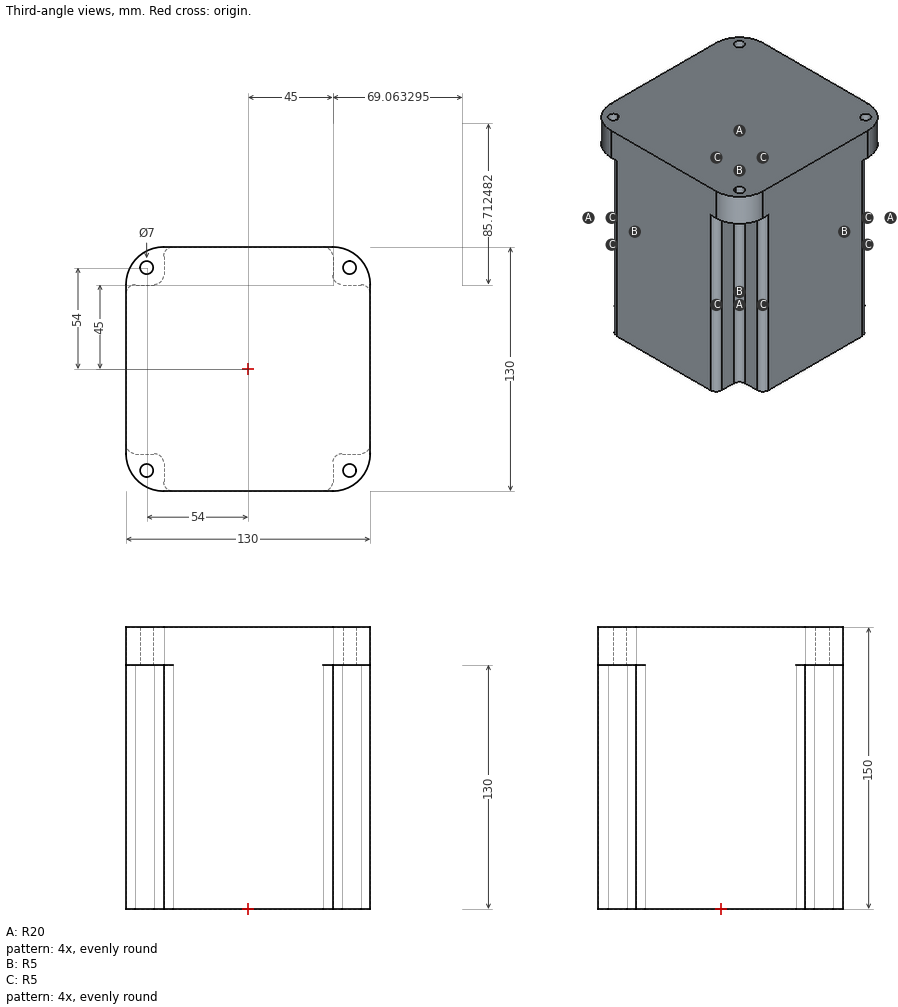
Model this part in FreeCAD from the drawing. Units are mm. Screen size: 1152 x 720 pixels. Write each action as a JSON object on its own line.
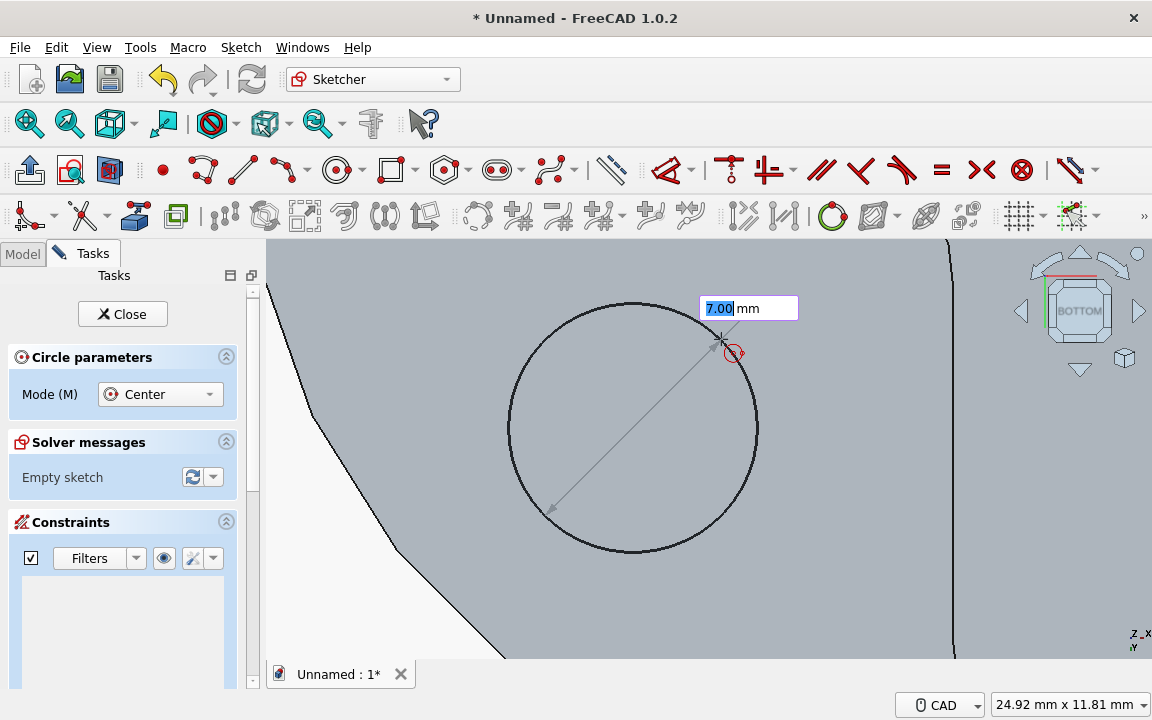
{"action": "type", "text": "7"}
{"action": "key", "text": "Return"}
{"action": "key", "text": "Escape"}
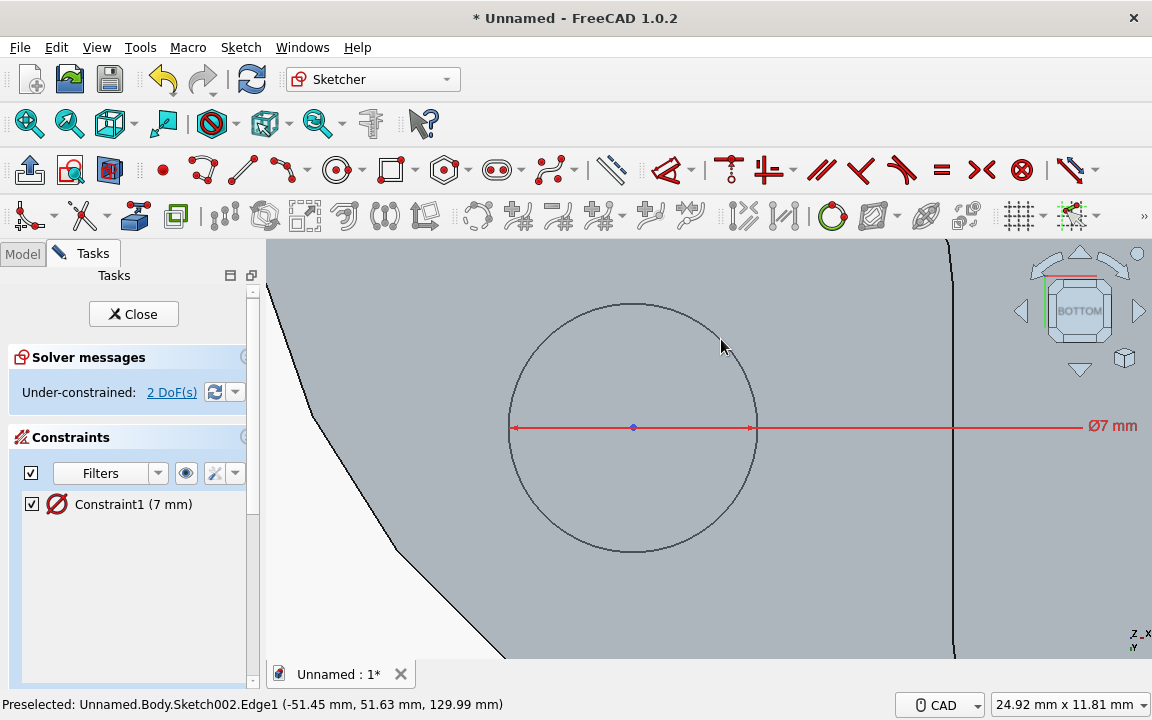
{"action": "key", "text": "d"}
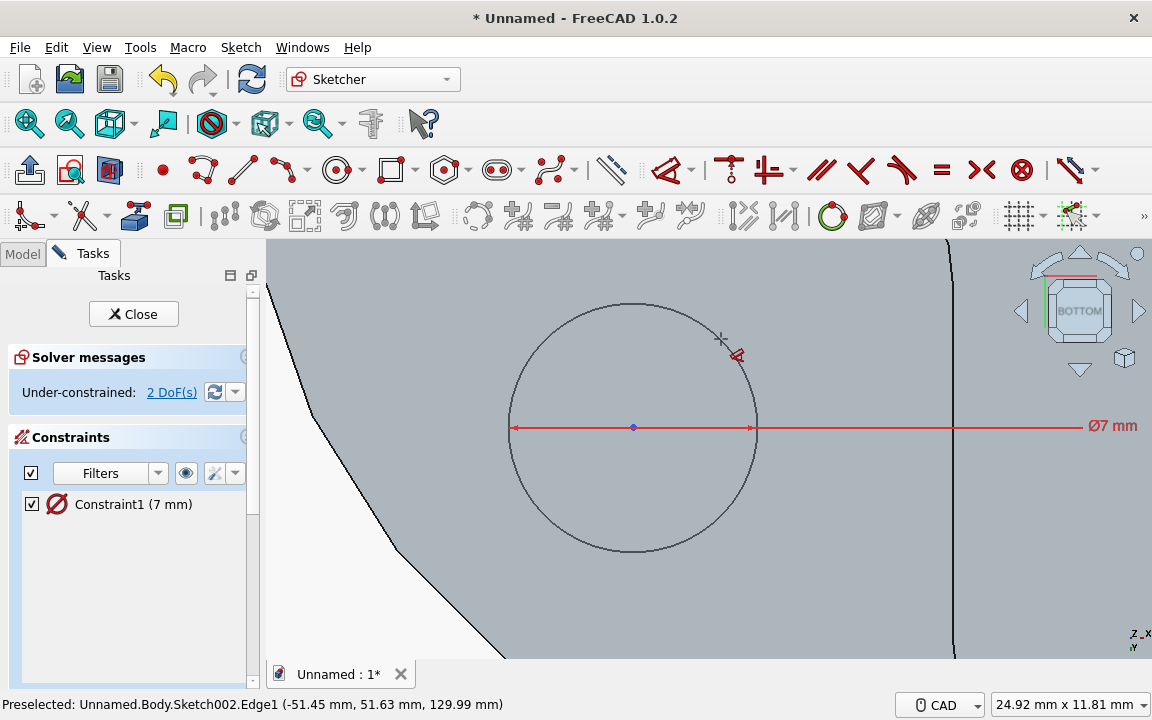
{"action": "left_click", "coordinate": [633, 428]}
{"action": "left_click", "coordinate": [810, 462]}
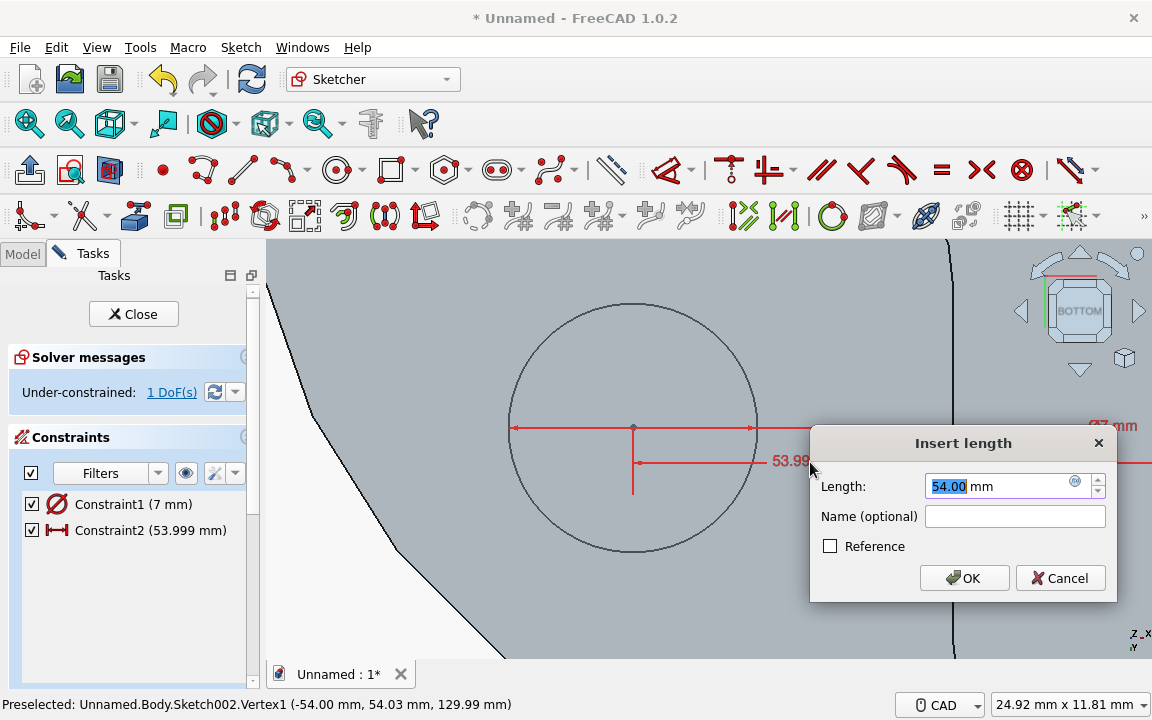
{"action": "type", "text": "54"}
{"action": "key", "text": "Return"}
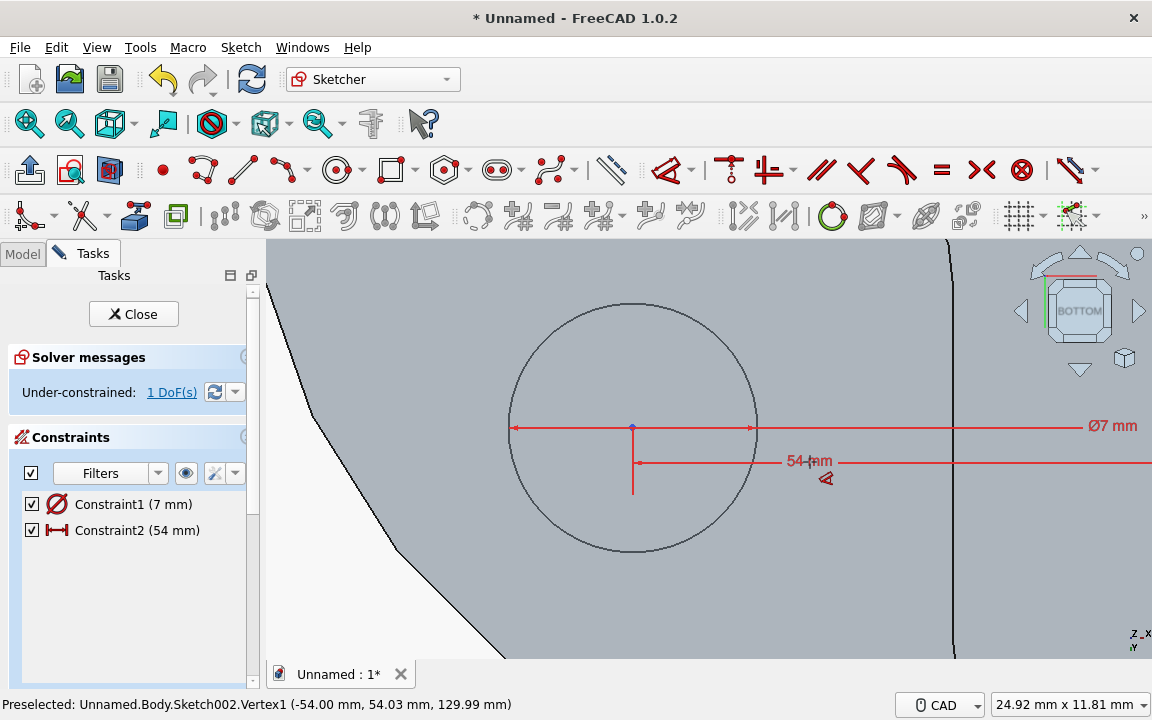
{"action": "left_click", "coordinate": [633, 428]}
{"action": "left_click", "coordinate": [599, 348]}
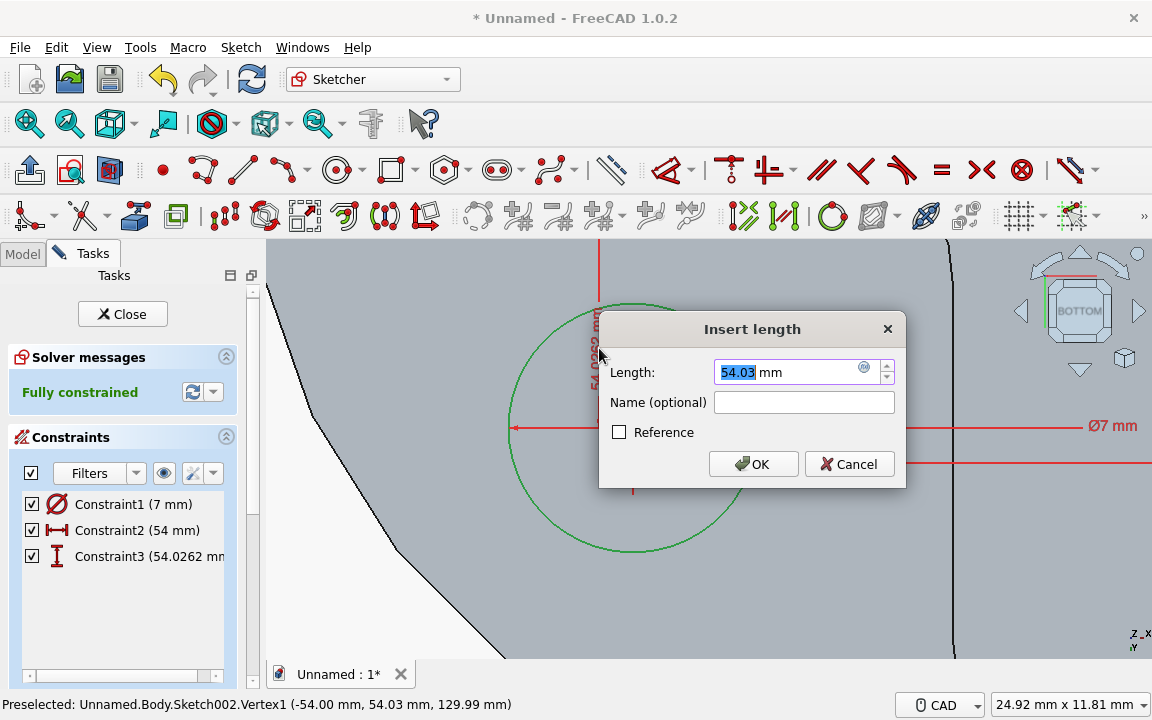
{"action": "type", "text": "54"}
{"action": "key", "text": "Return"}
{"action": "key", "text": "Escape"}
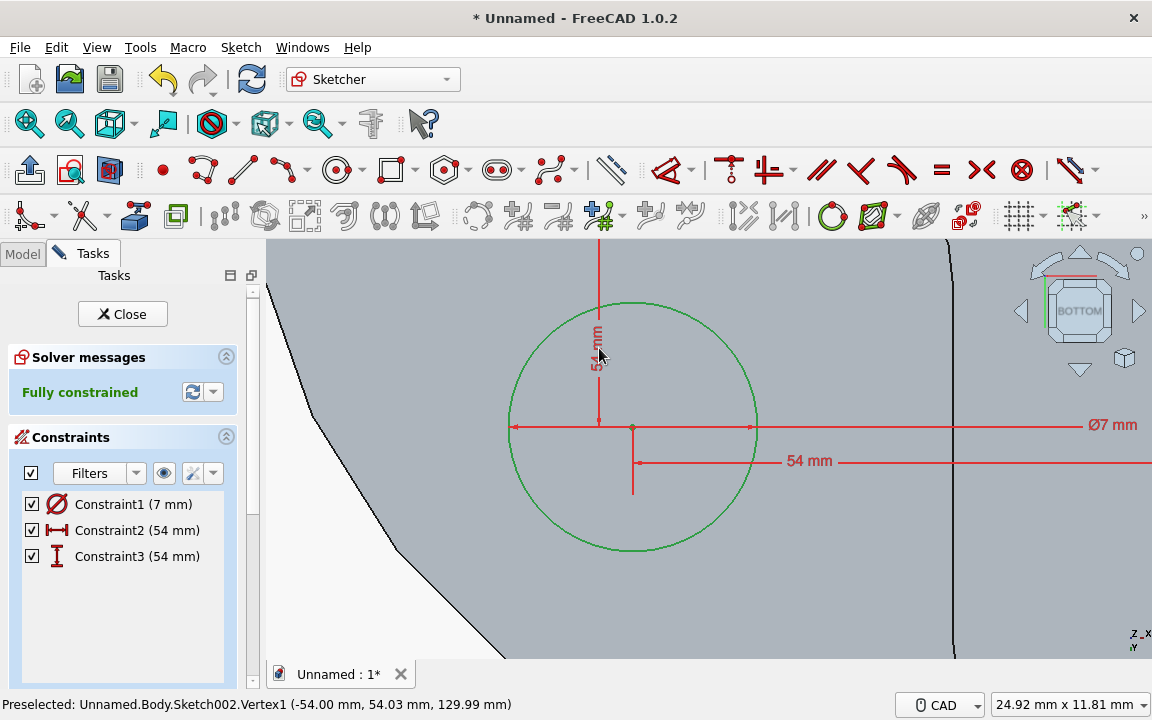
{"action": "left_click", "coordinate": [123, 314]}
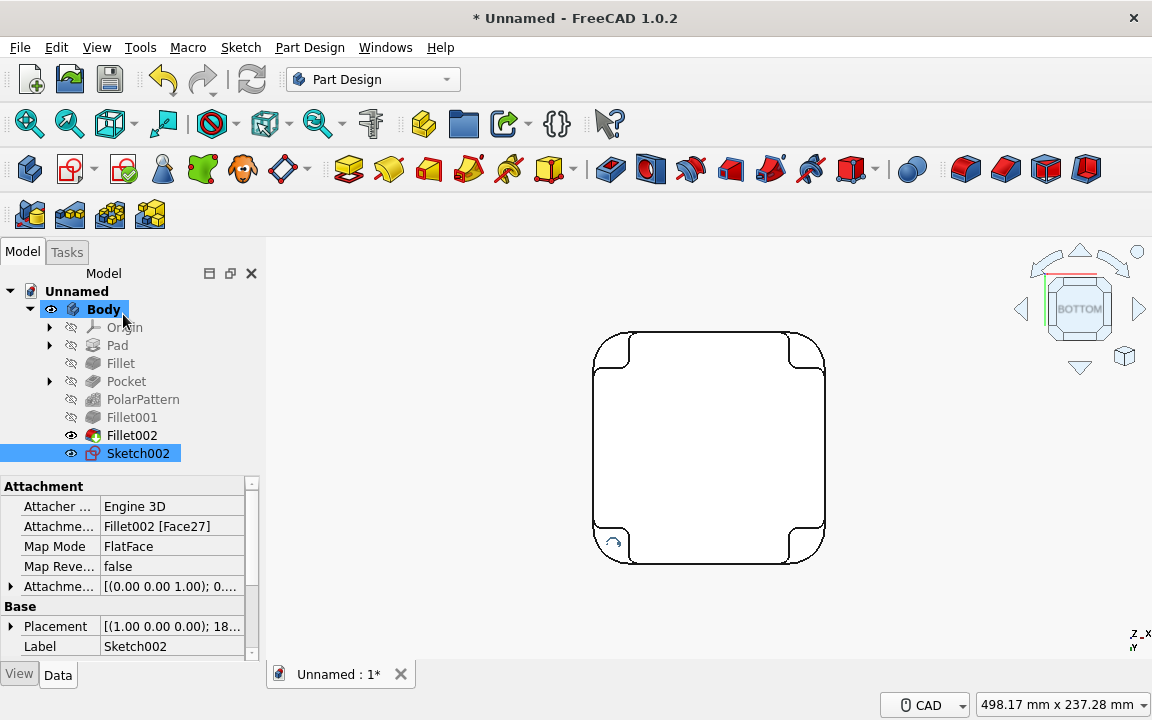
{"action": "left_click", "coordinate": [612, 170]}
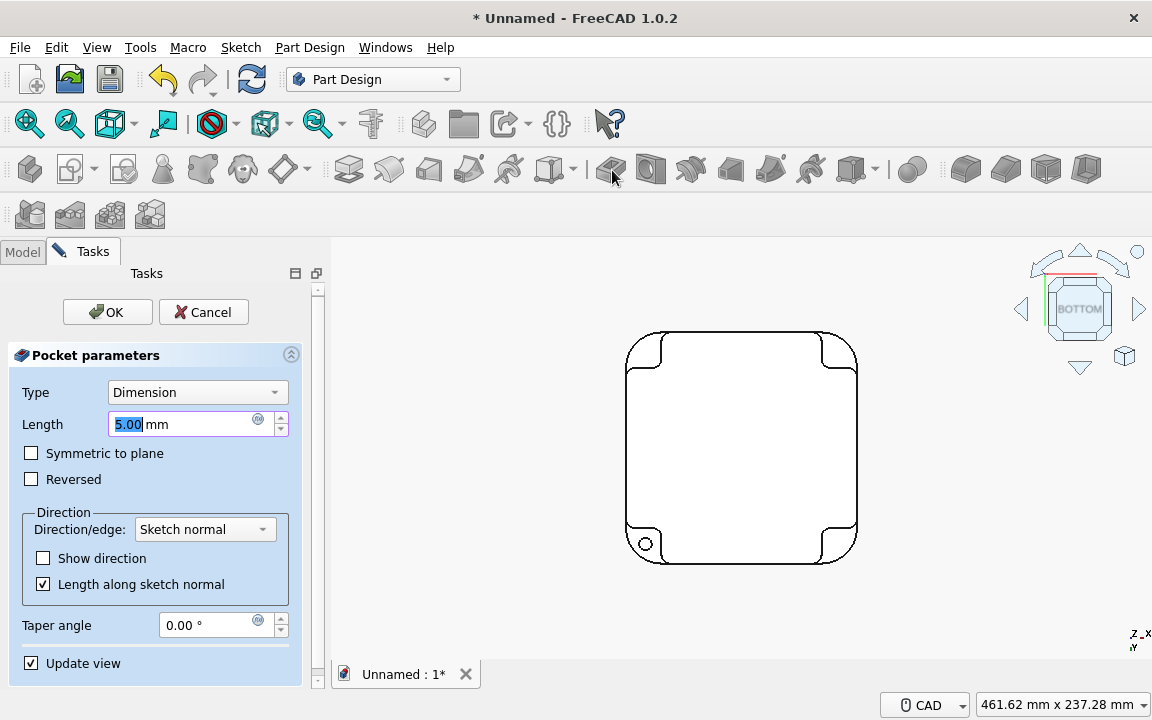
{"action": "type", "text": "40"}
{"action": "key", "text": "Tab"}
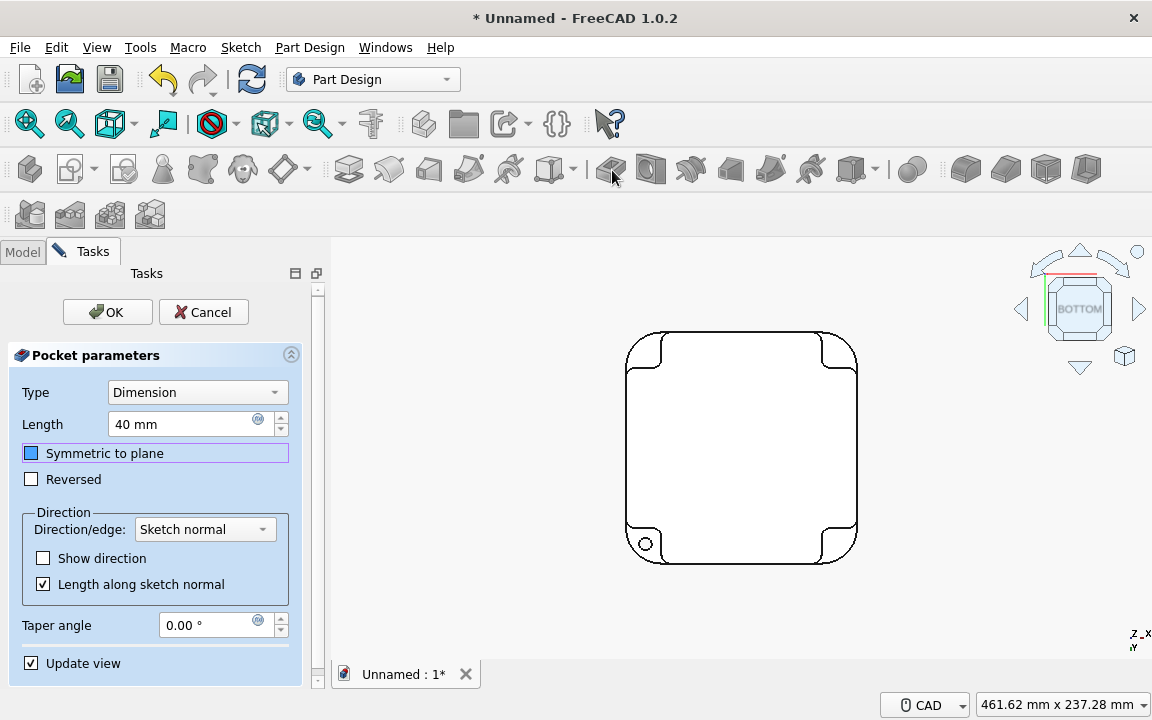
{"action": "left_click", "coordinate": [108, 312]}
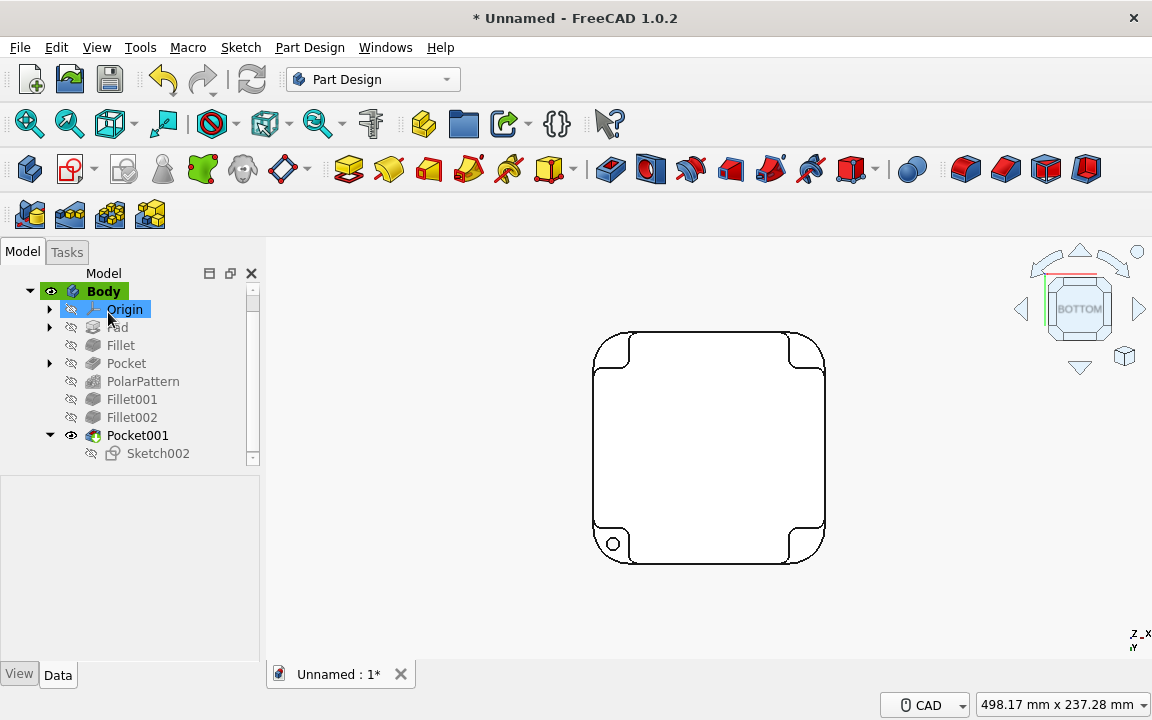
{"action": "left_click", "coordinate": [116, 435]}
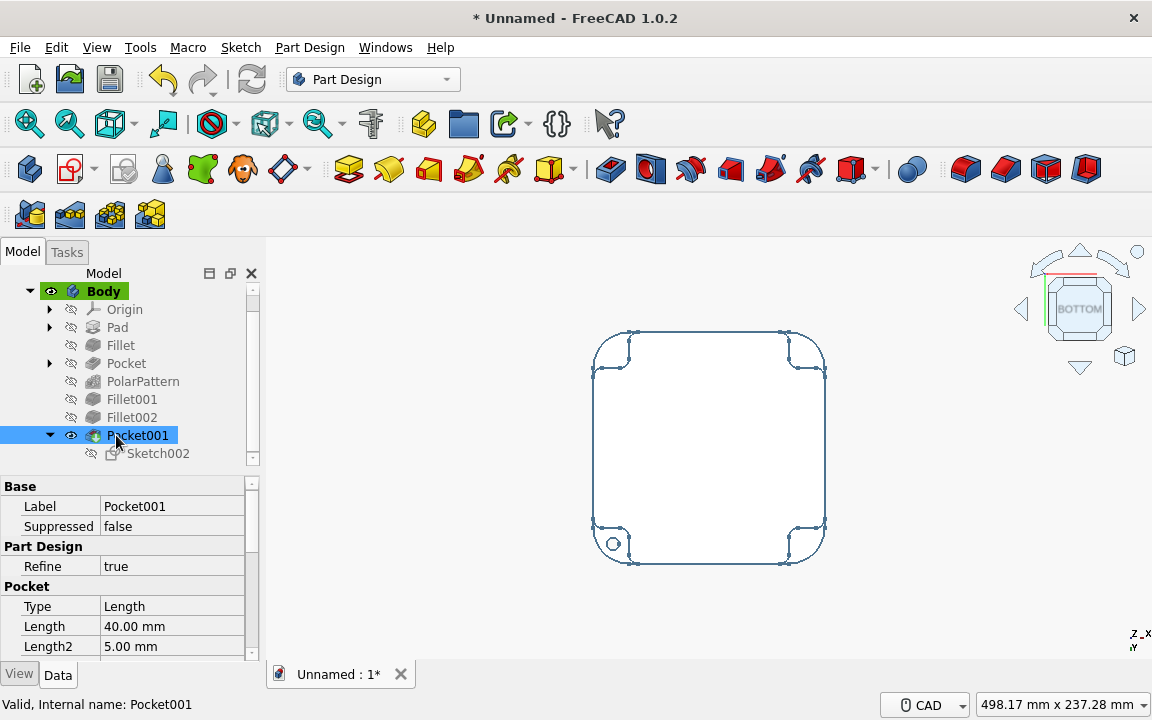
{"action": "left_click", "coordinate": [110, 214]}